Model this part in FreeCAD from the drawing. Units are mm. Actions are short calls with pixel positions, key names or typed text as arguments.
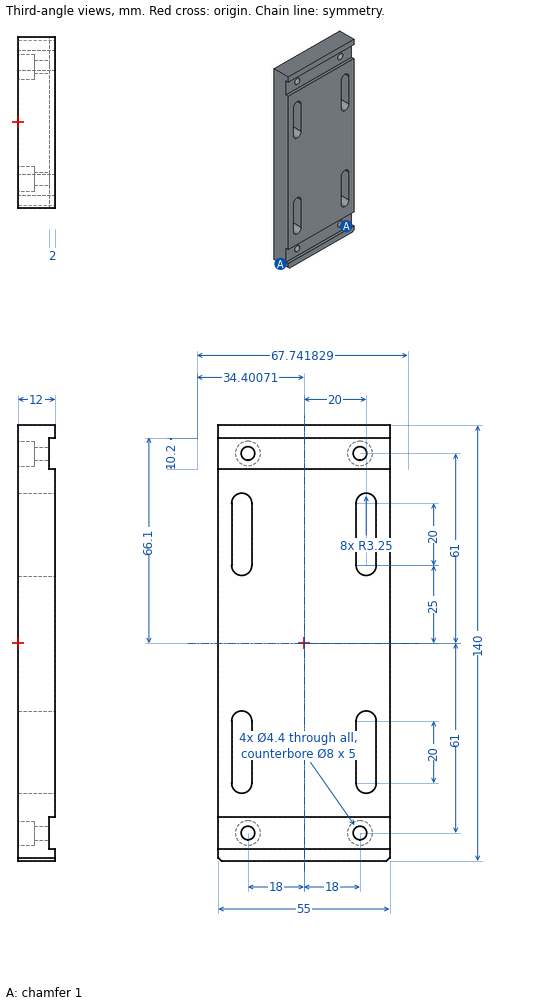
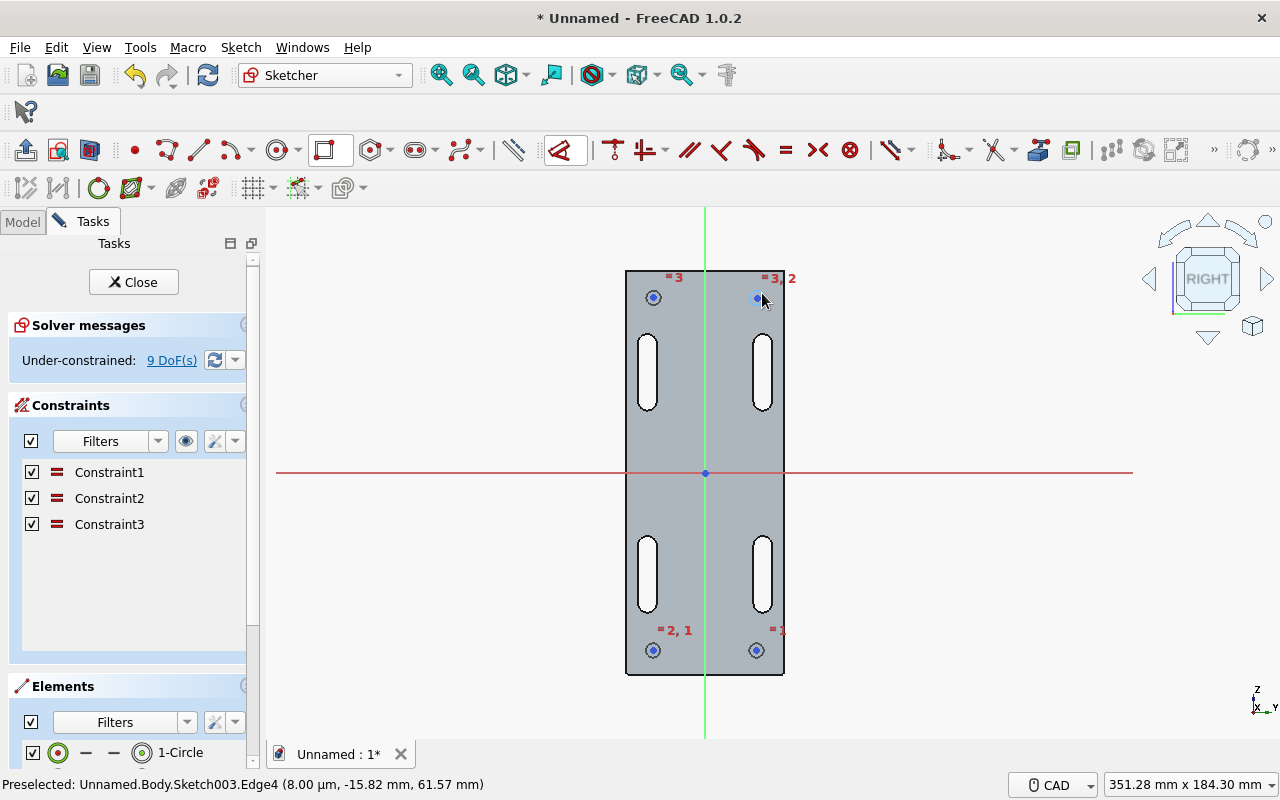
click(757, 651)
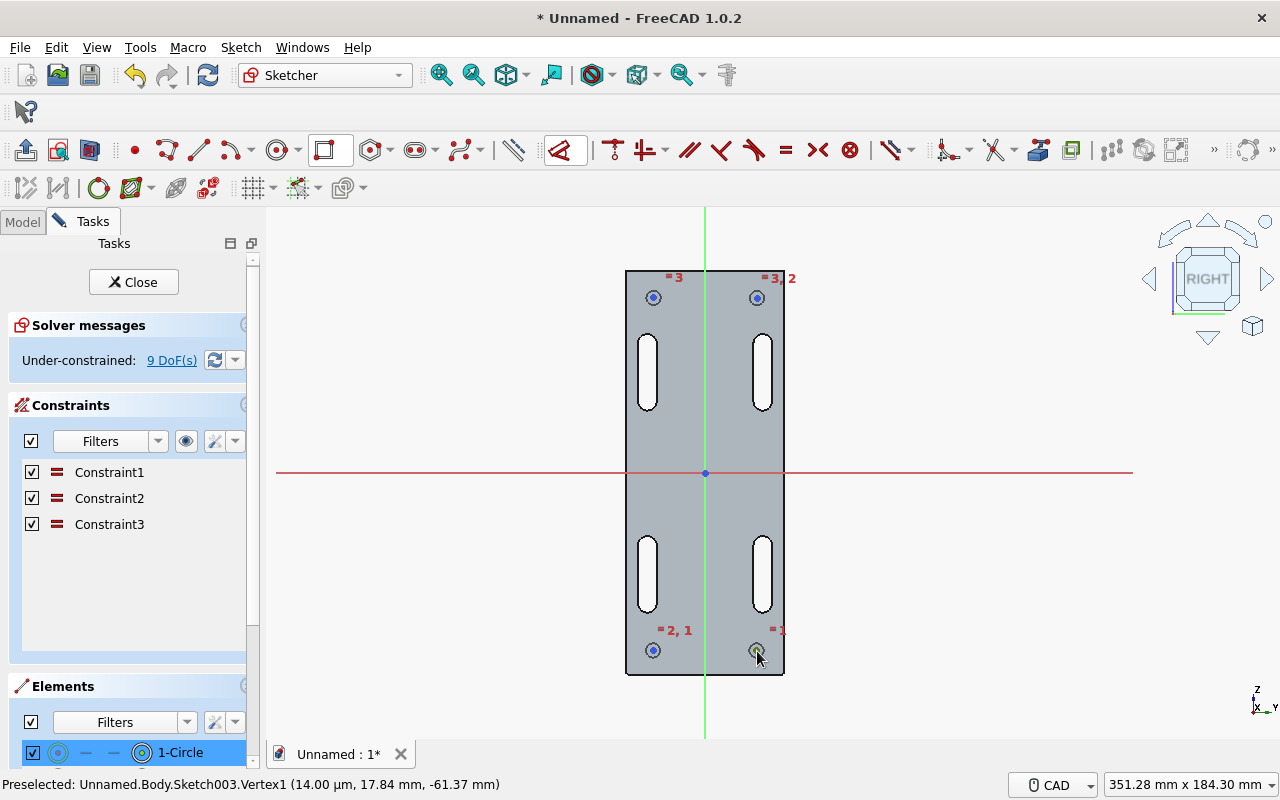
click(653, 650)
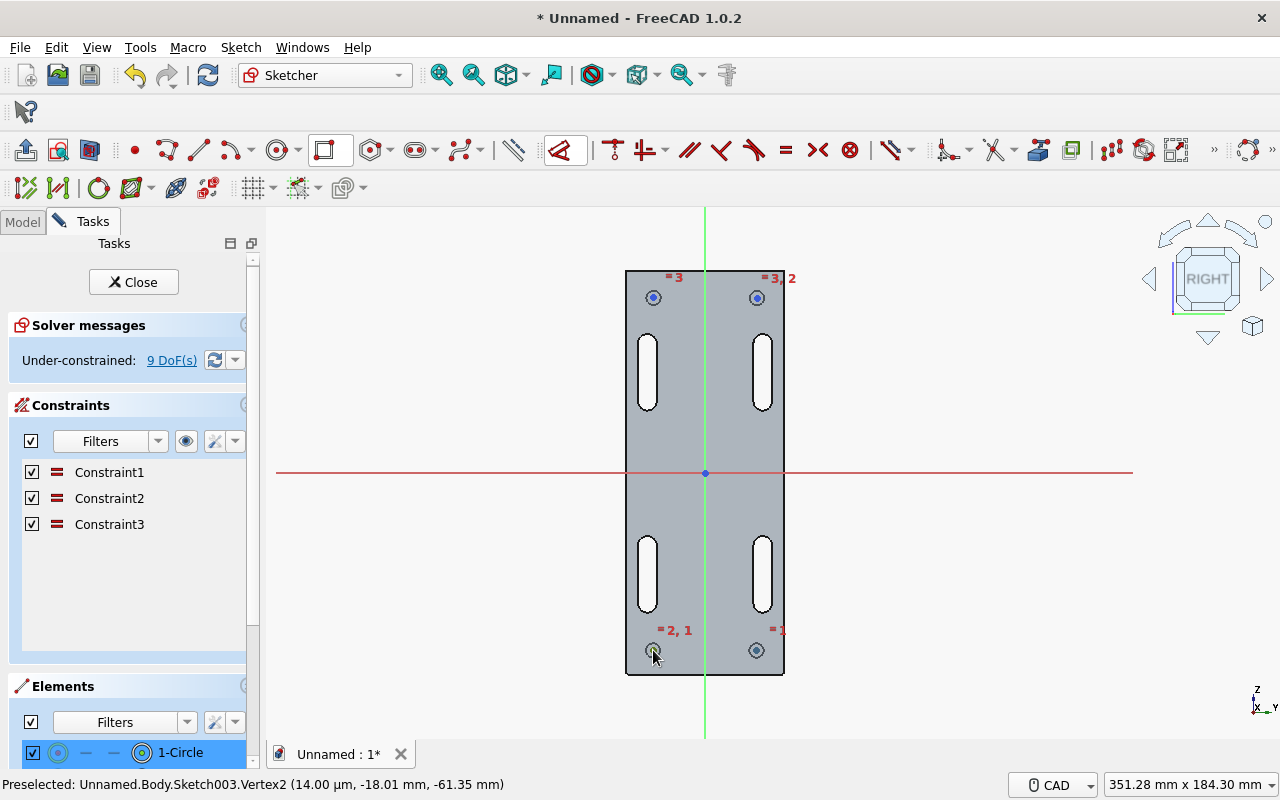
key(h)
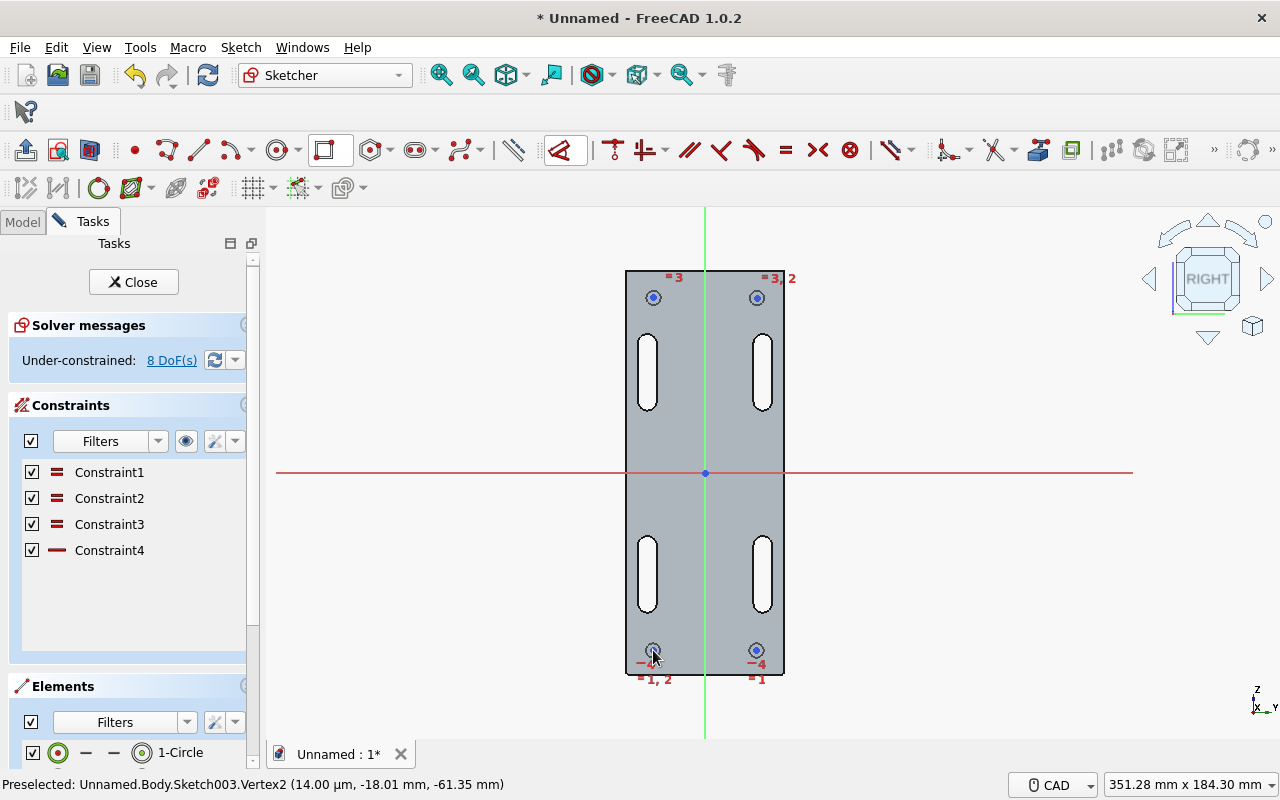
click(757, 651)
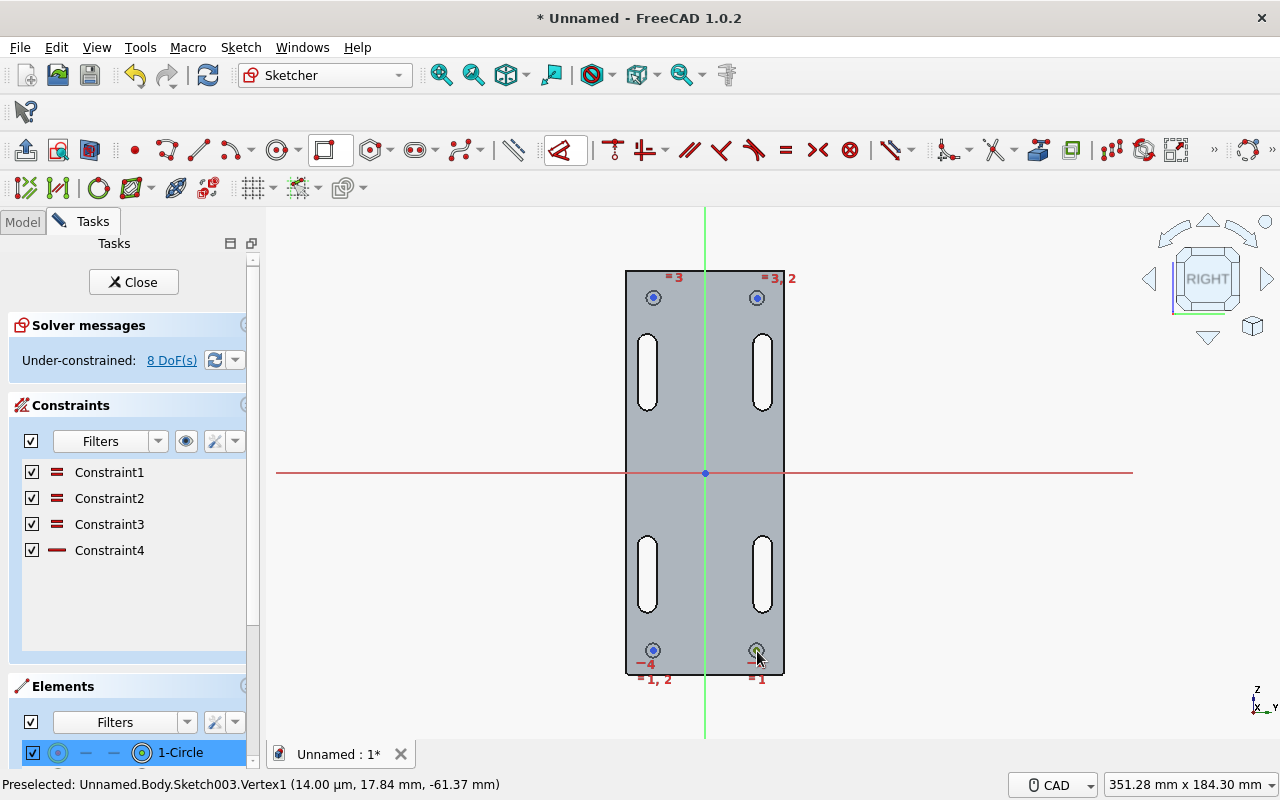
click(757, 298)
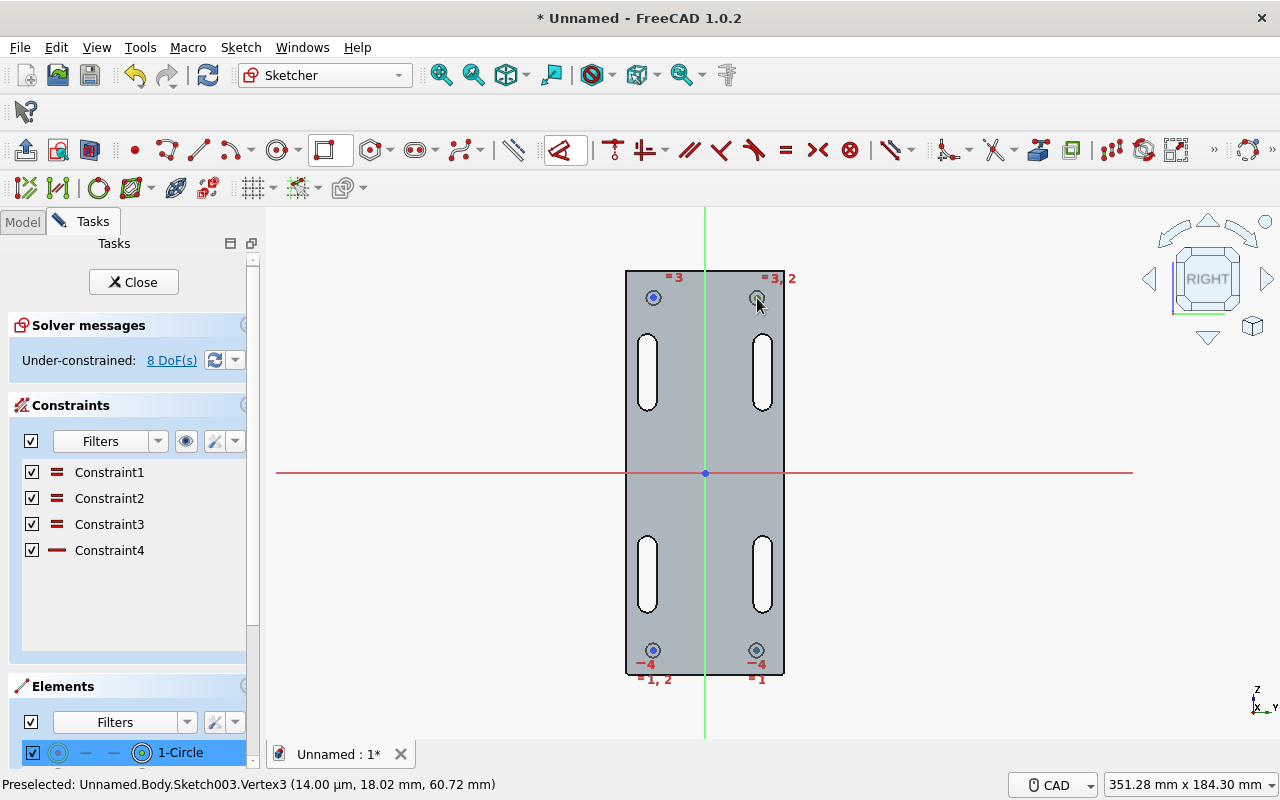
key(v)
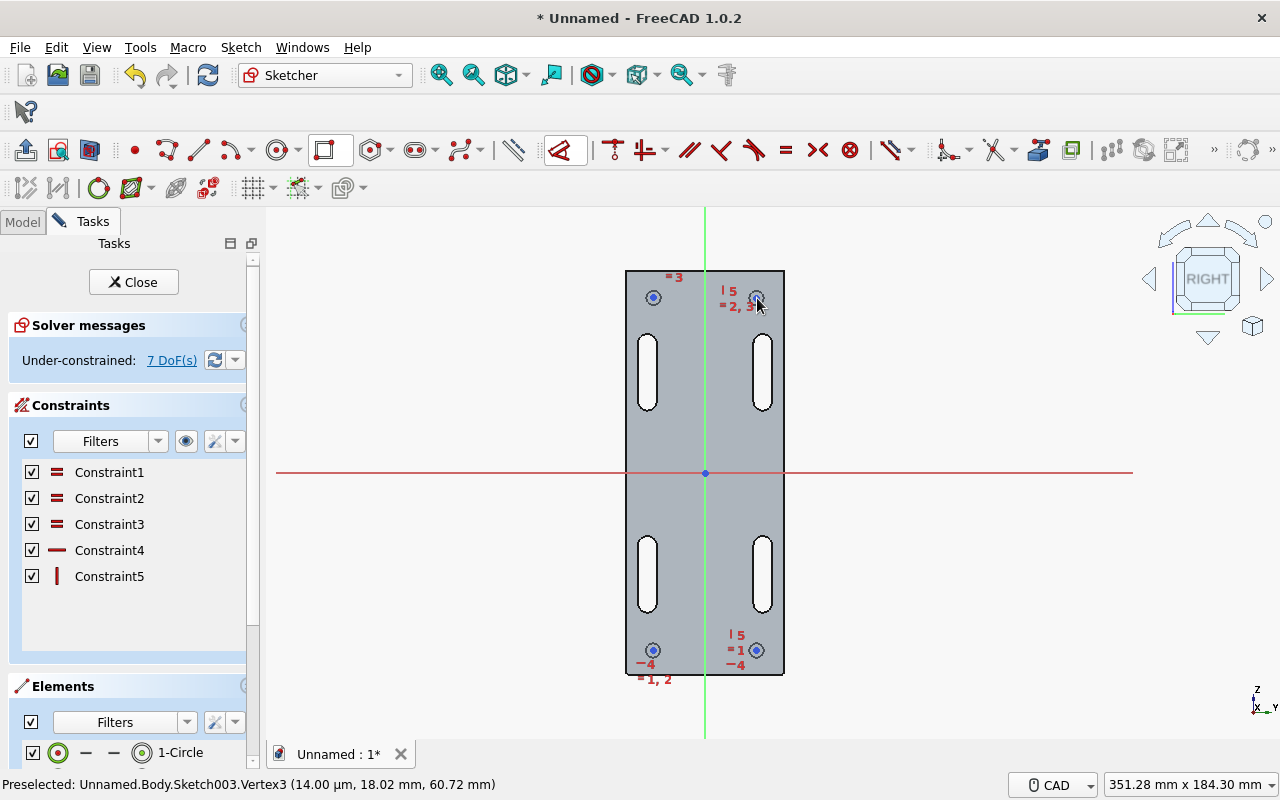
click(653, 651)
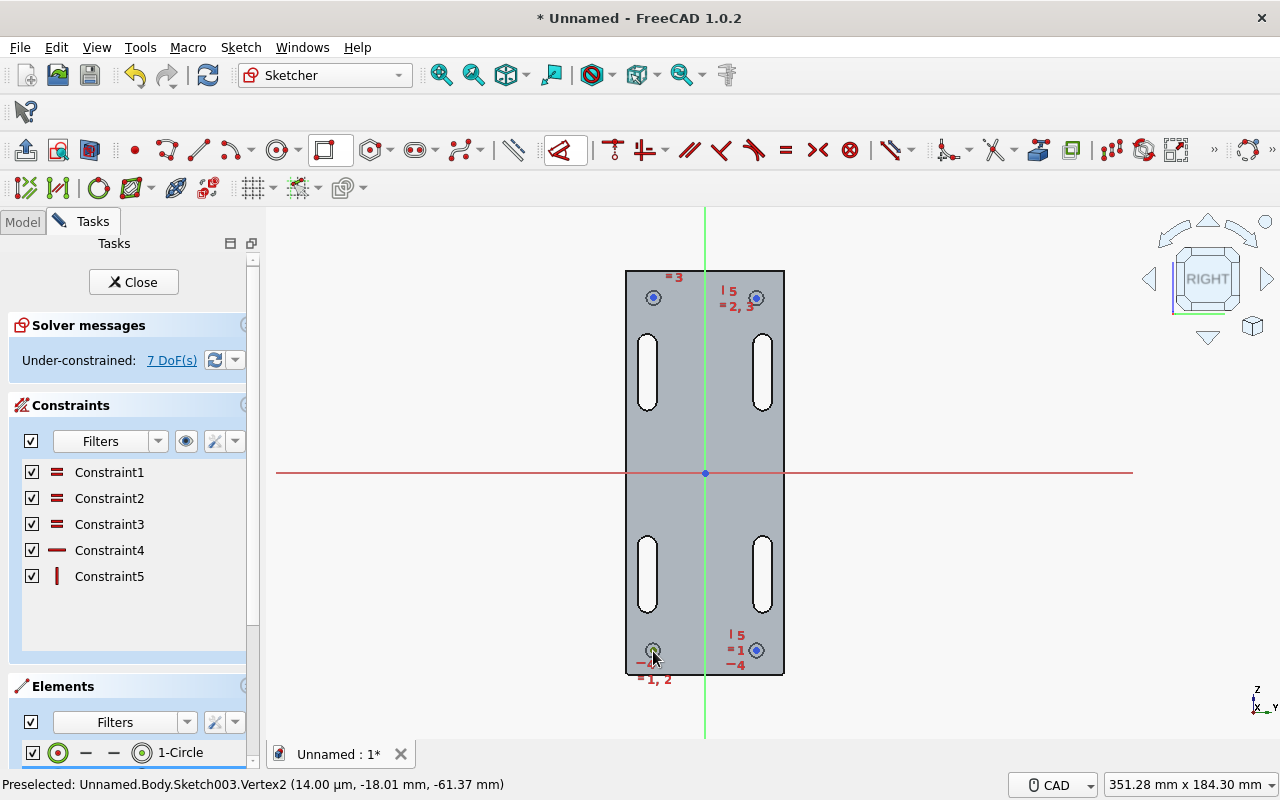
click(654, 298)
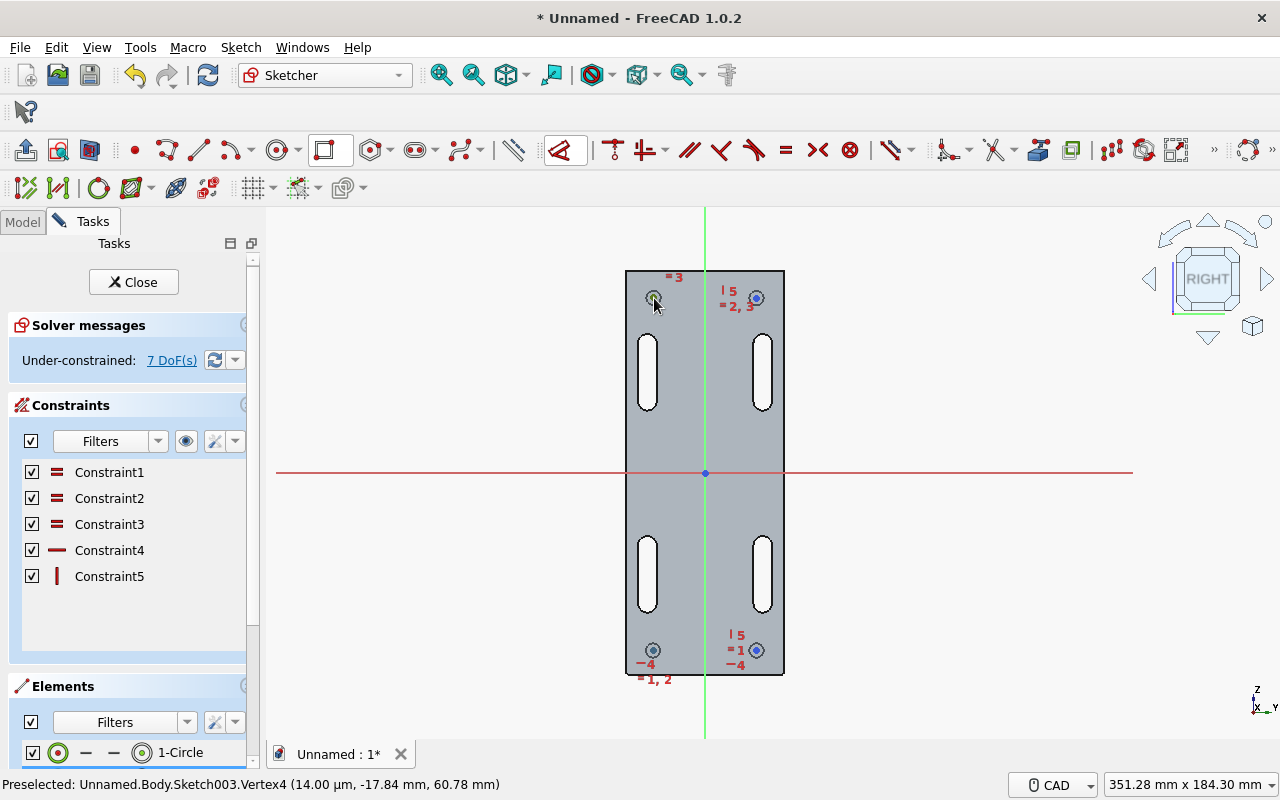
click(668, 150)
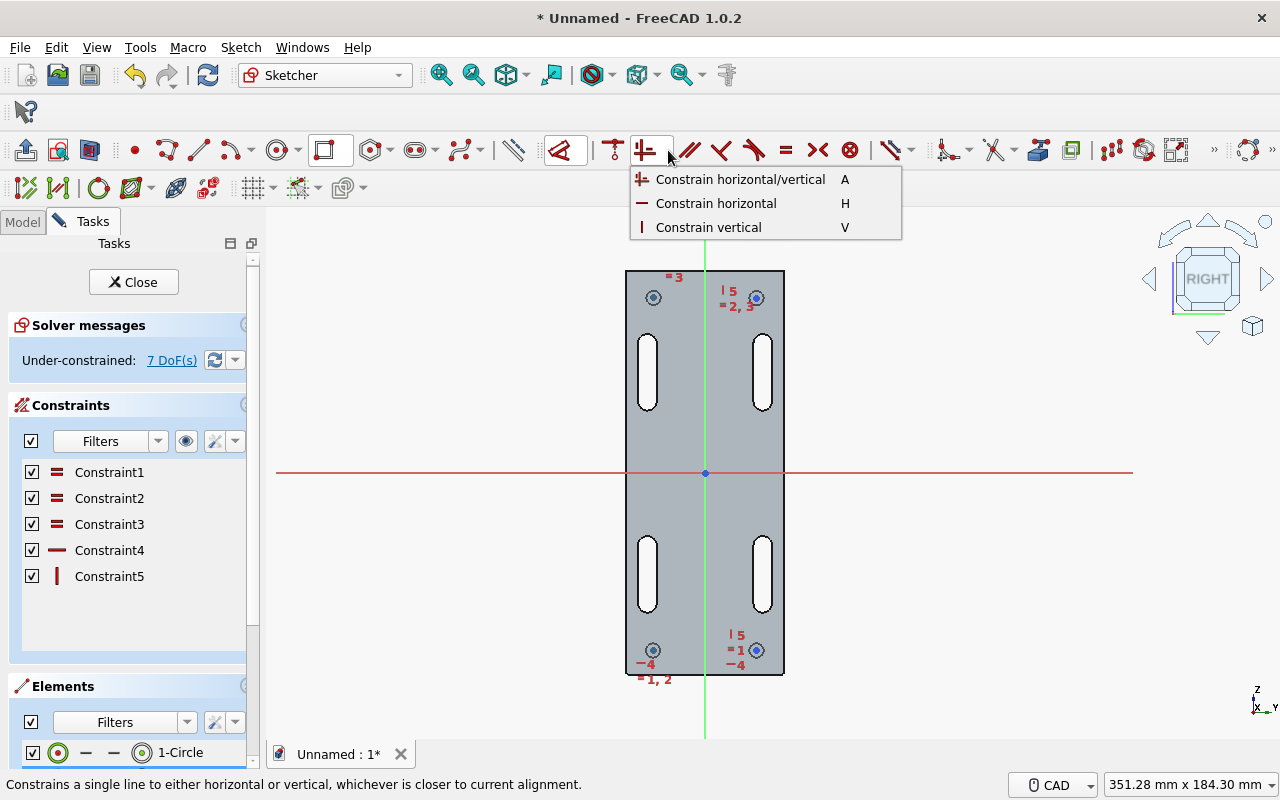
click(766, 227)